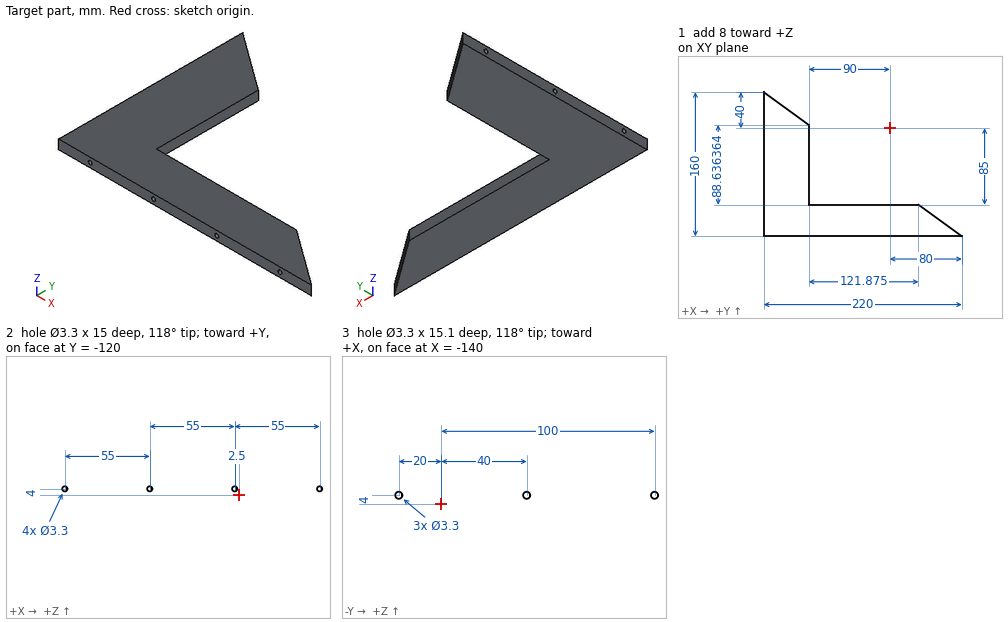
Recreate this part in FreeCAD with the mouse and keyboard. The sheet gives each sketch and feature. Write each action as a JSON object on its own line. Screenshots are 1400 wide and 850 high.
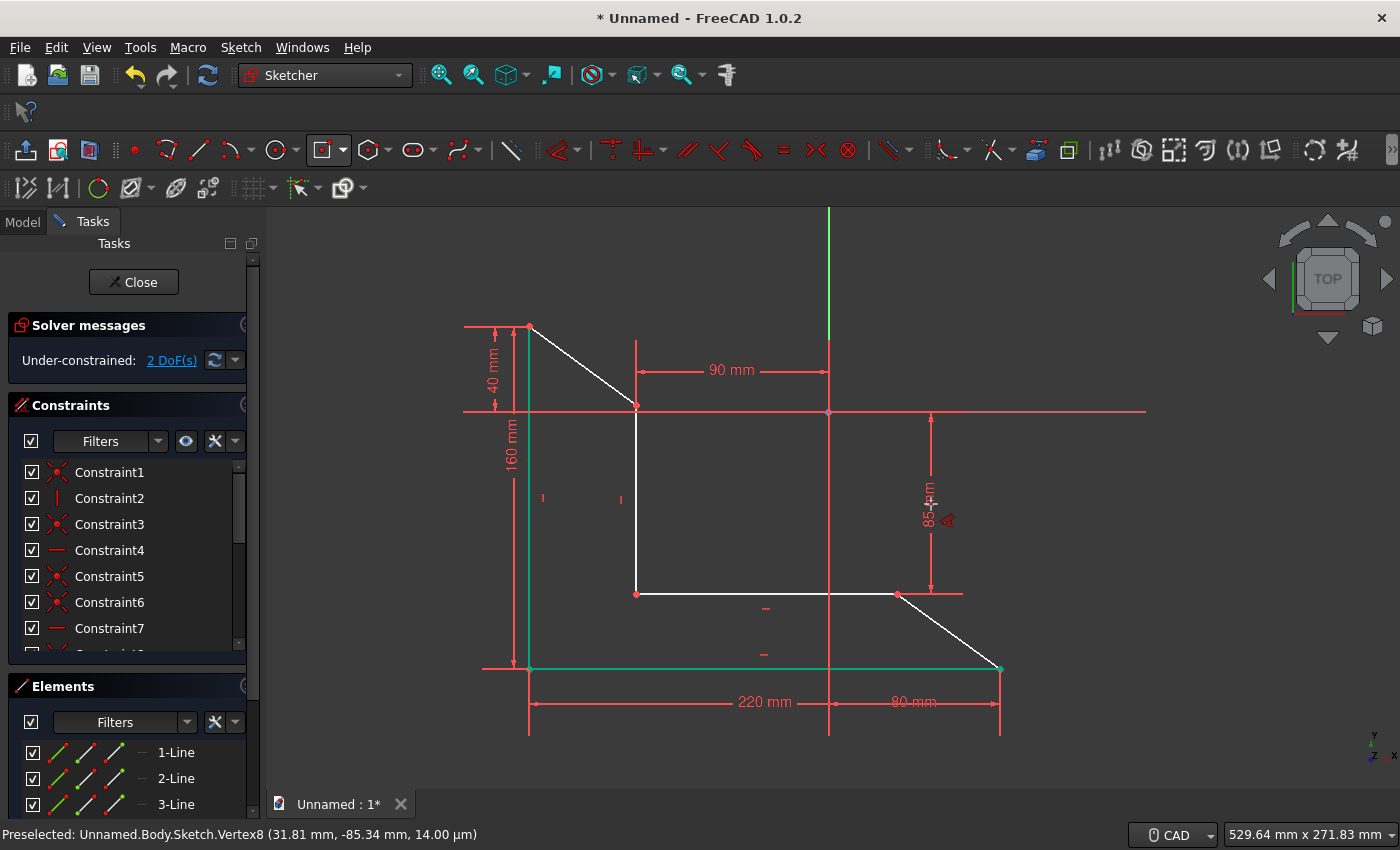
{"action": "scroll", "coordinate": [819, 594], "scroll_direction": "up", "scroll_amount": 2}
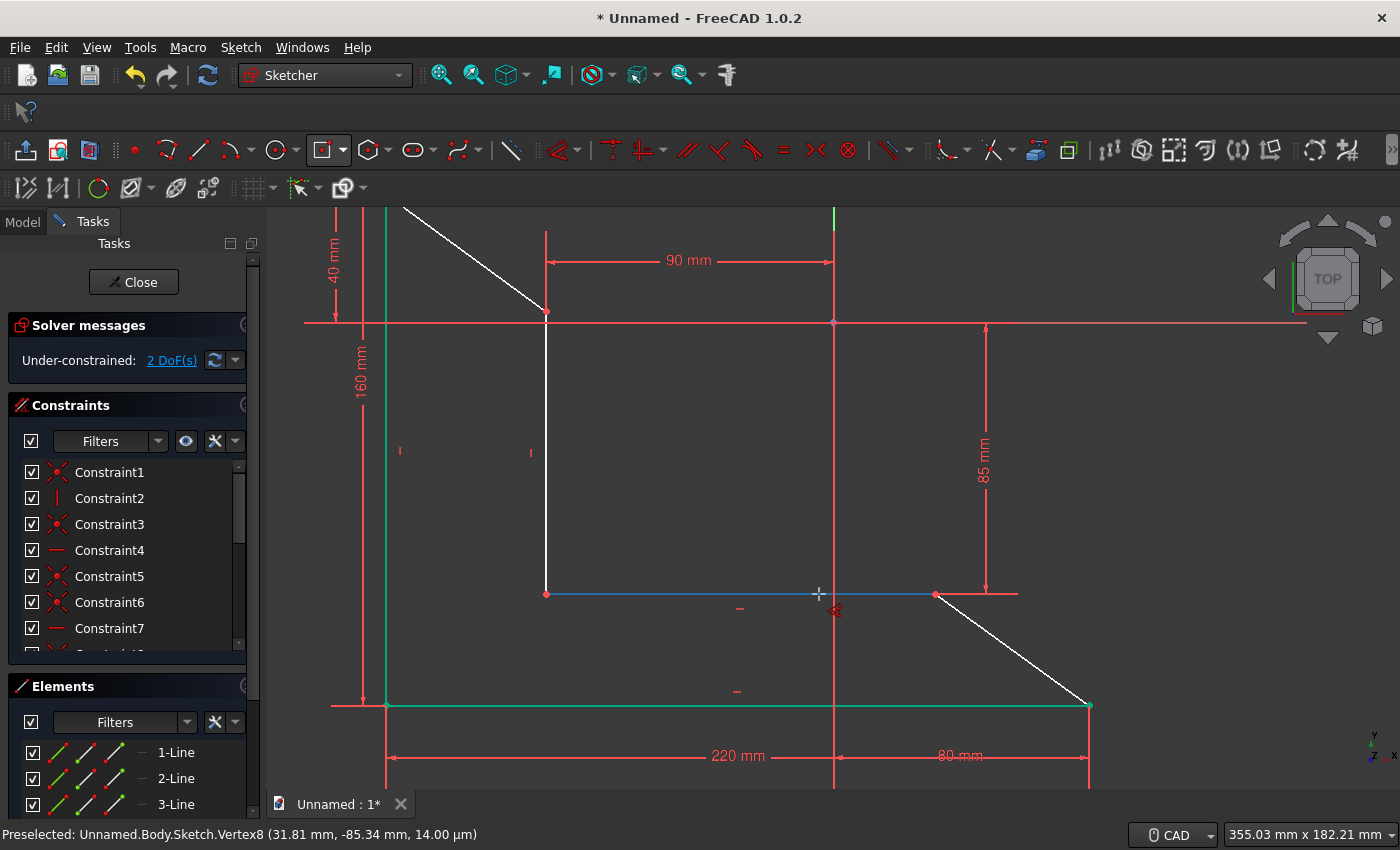
{"action": "left_click", "coordinate": [818, 594]}
{"action": "left_click", "coordinate": [741, 628]}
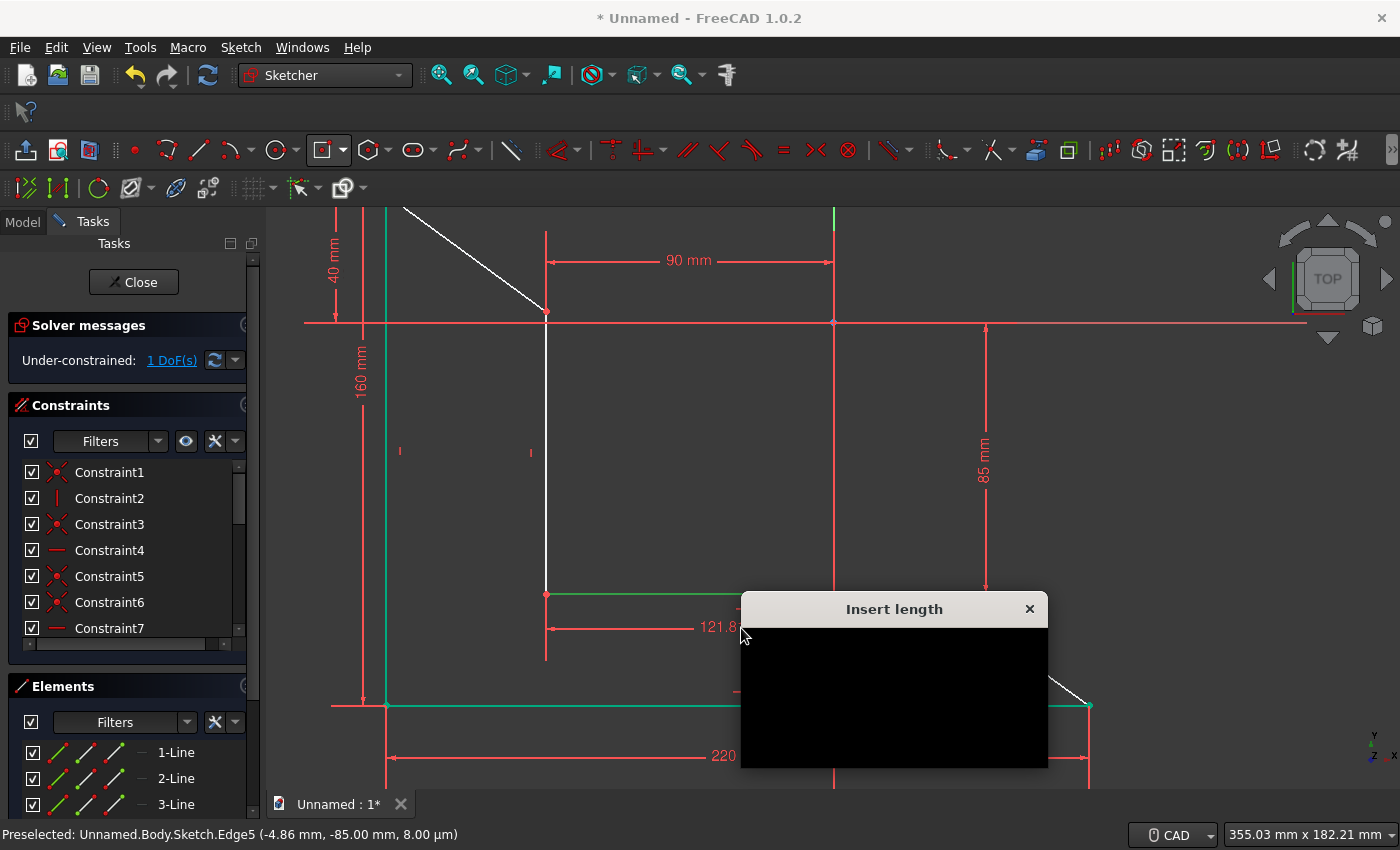
{"action": "type", "text": "121.875"}
{"action": "key", "text": "Return"}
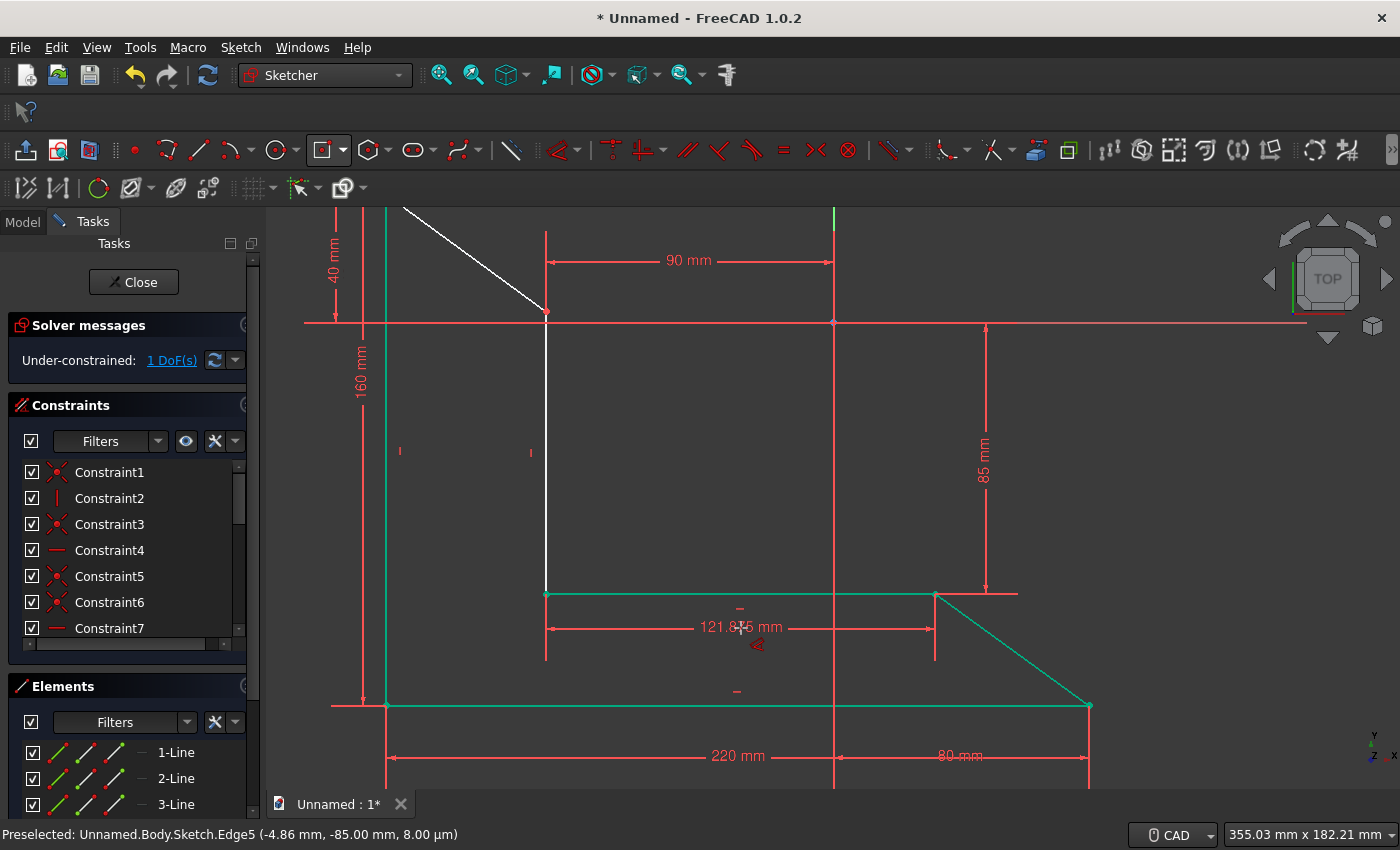
{"action": "left_click", "coordinate": [546, 509]}
{"action": "left_click", "coordinate": [512, 453]}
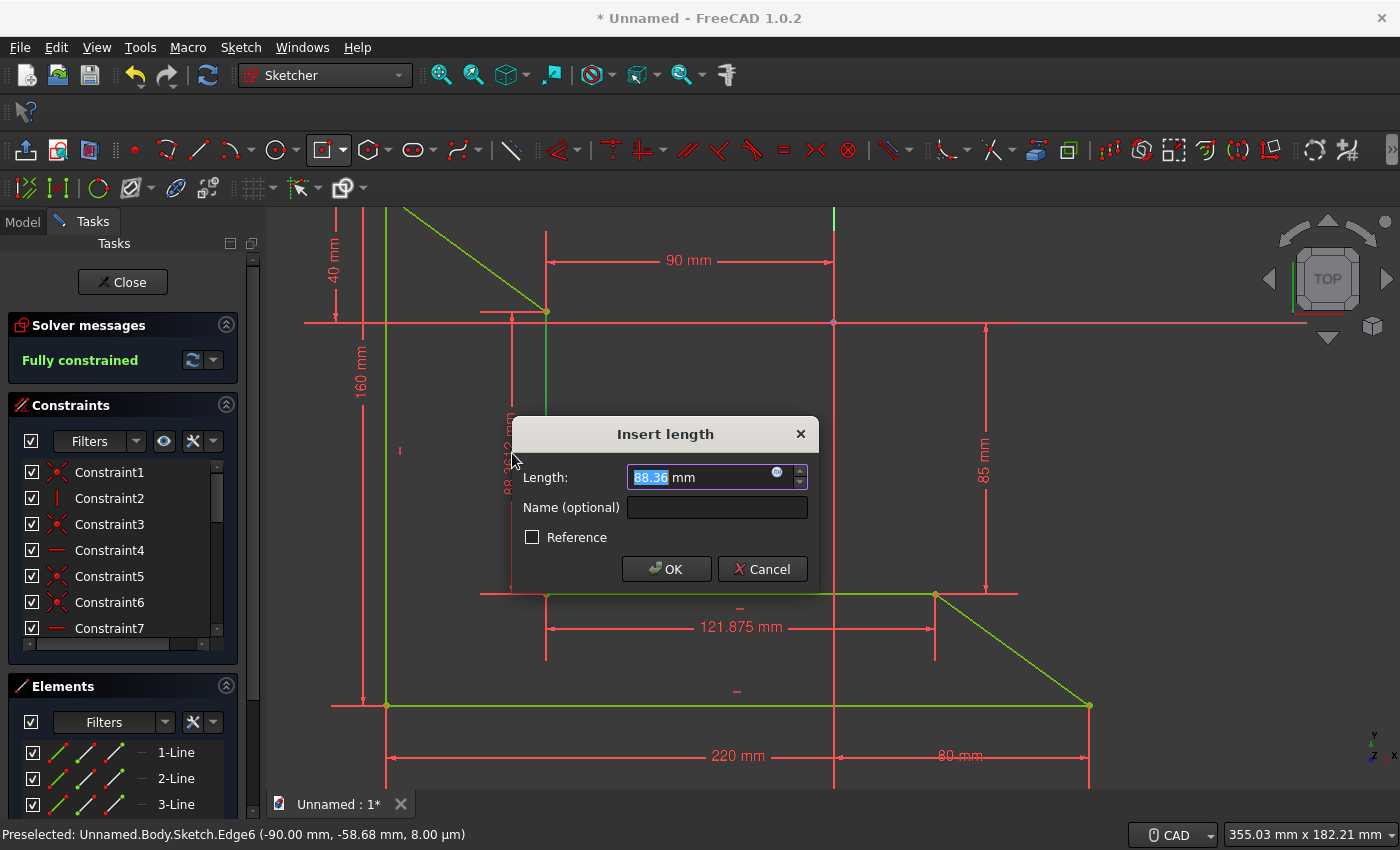
{"action": "type", "text": "88.636364"}
{"action": "key", "text": "Return"}
{"action": "key", "text": "Escape"}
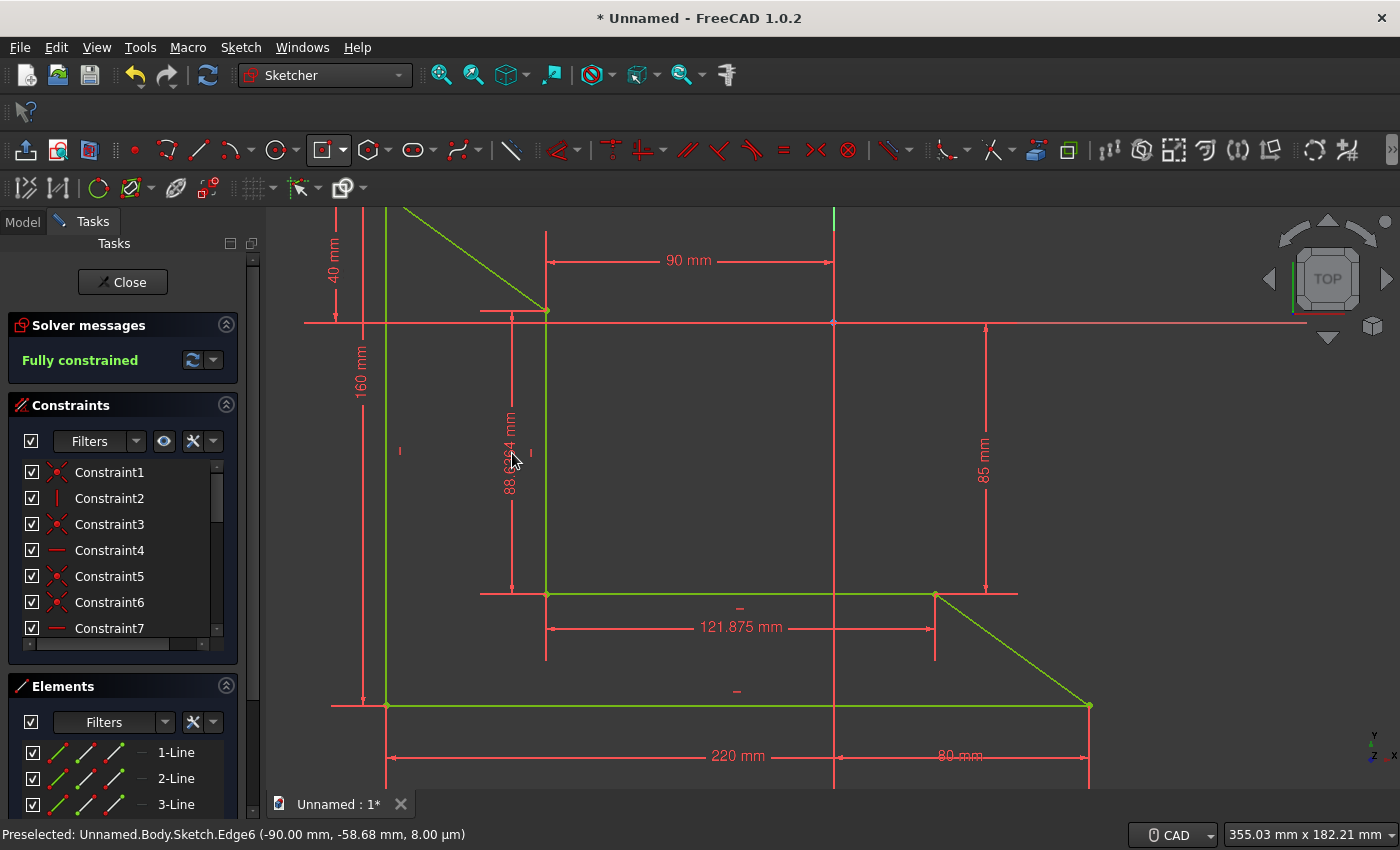
{"action": "left_click", "coordinate": [123, 282]}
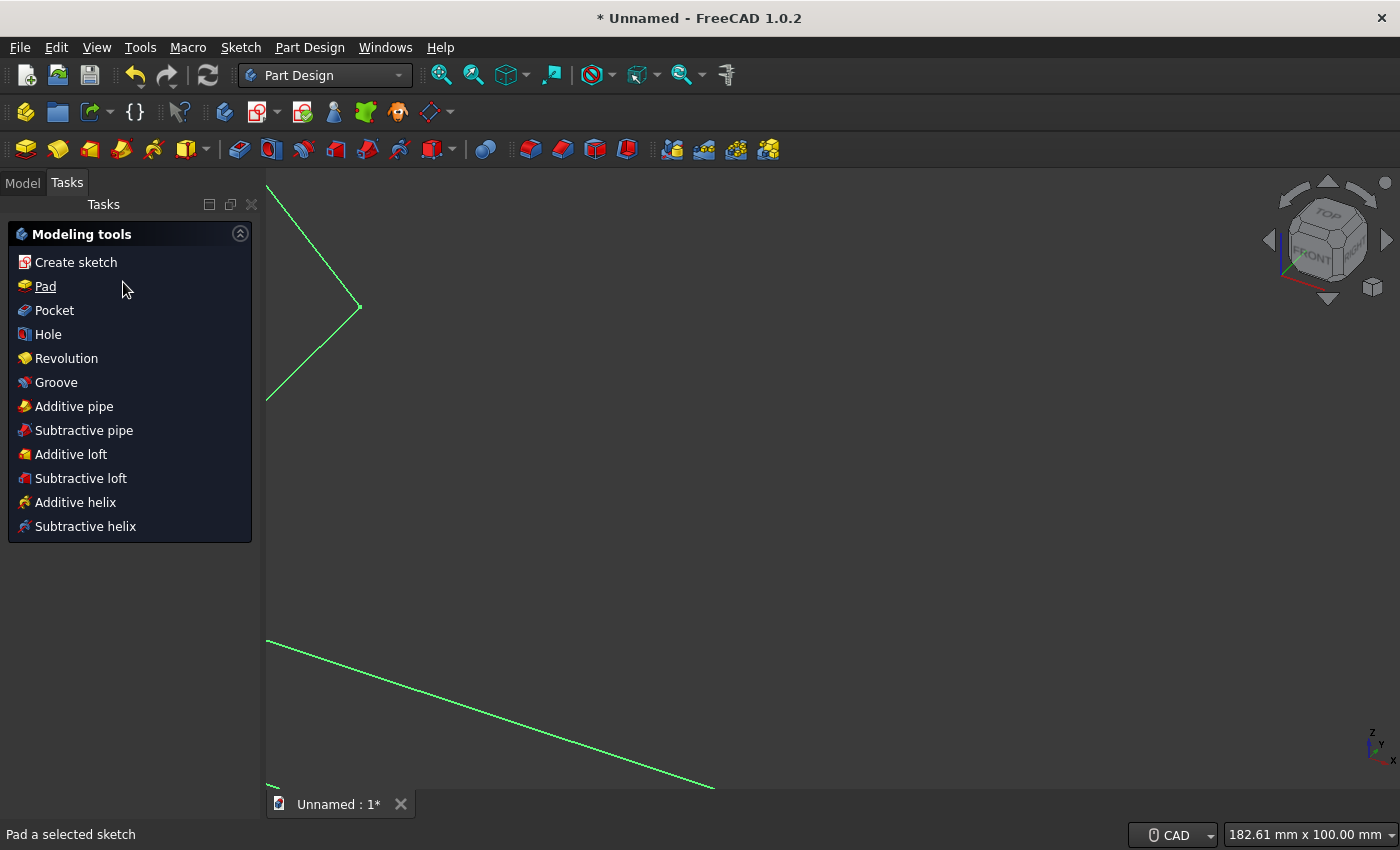
{"action": "left_click", "coordinate": [26, 150]}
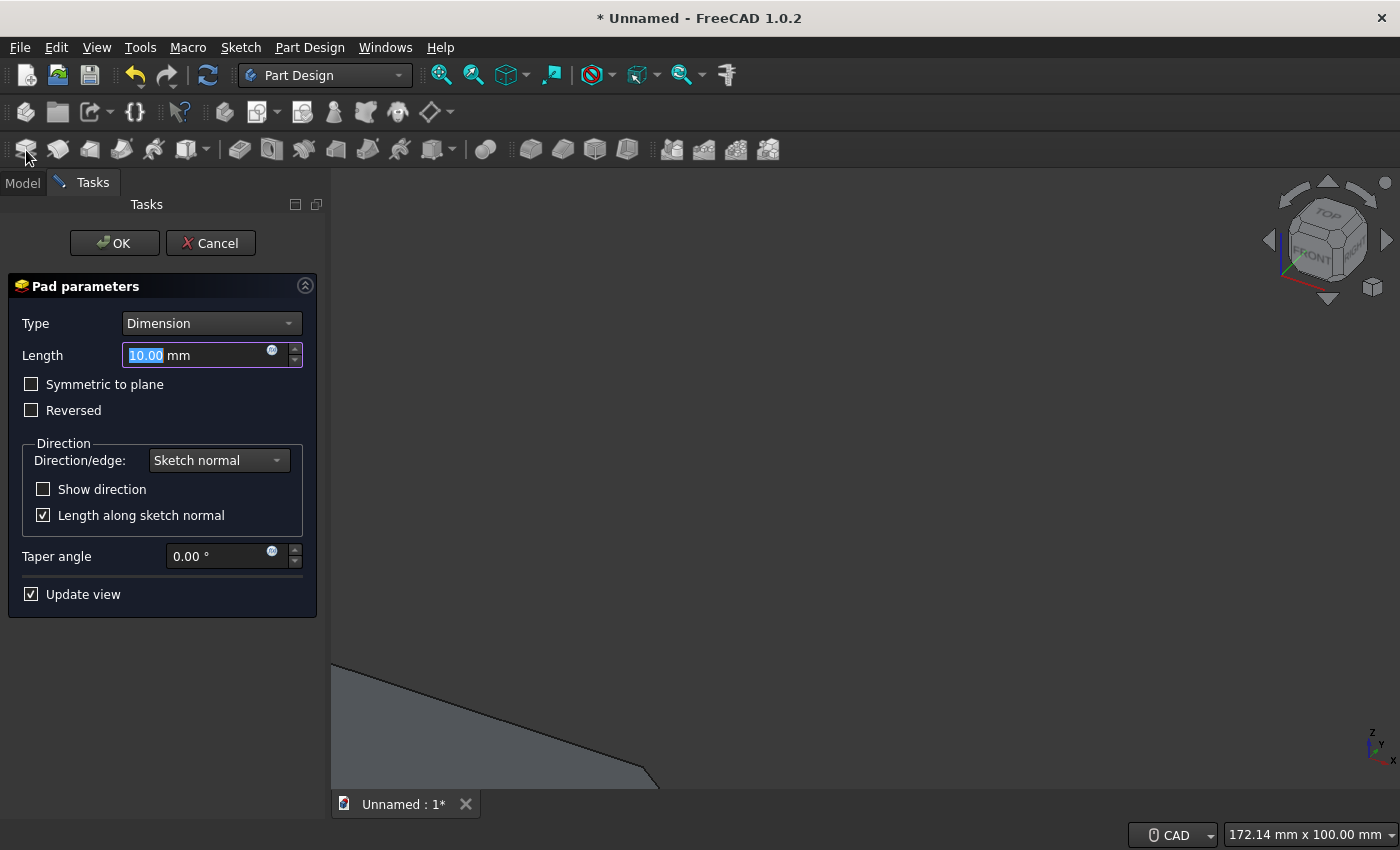
{"action": "type", "text": "8"}
{"action": "key", "text": "Tab"}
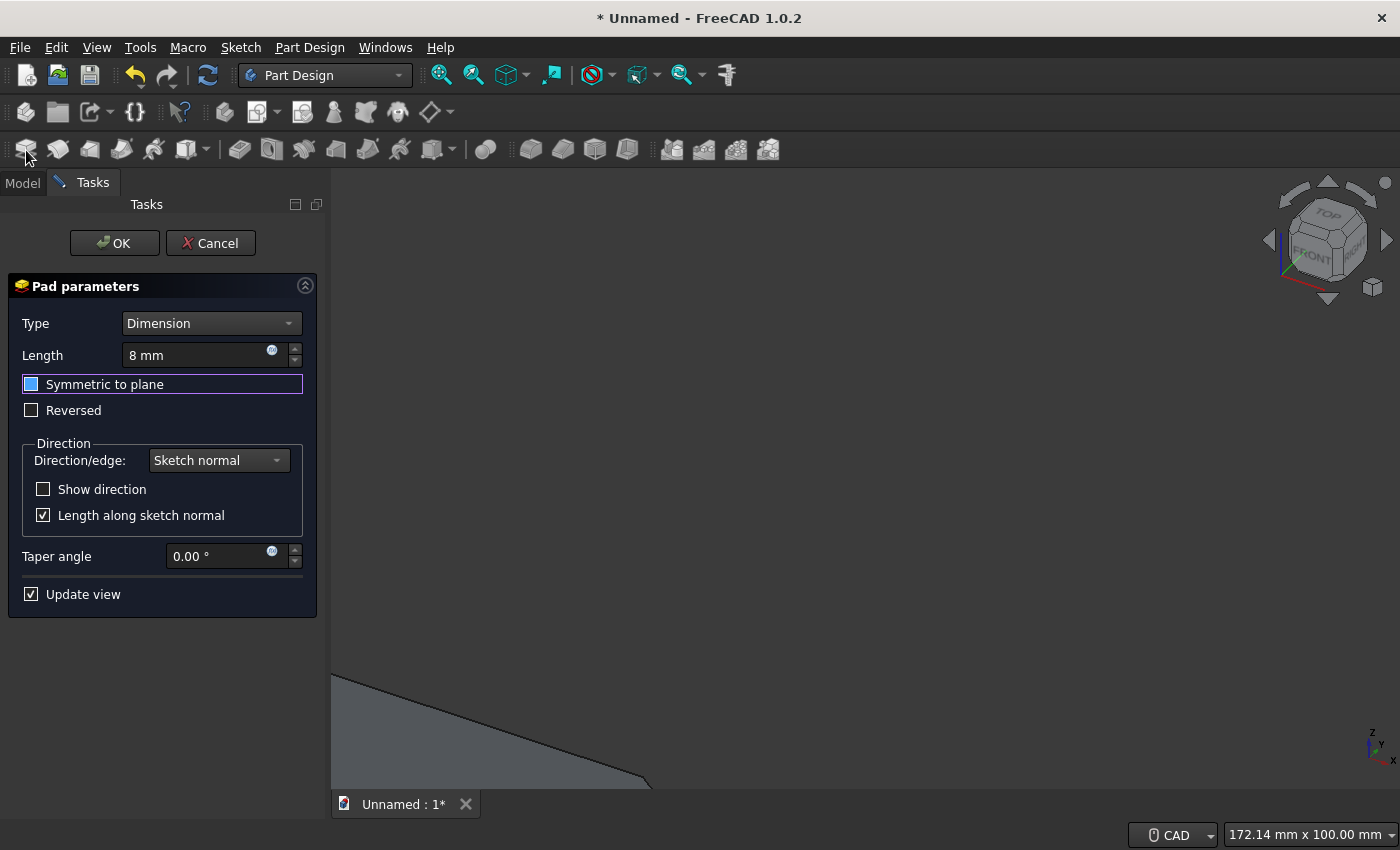
{"action": "left_click", "coordinate": [115, 243]}